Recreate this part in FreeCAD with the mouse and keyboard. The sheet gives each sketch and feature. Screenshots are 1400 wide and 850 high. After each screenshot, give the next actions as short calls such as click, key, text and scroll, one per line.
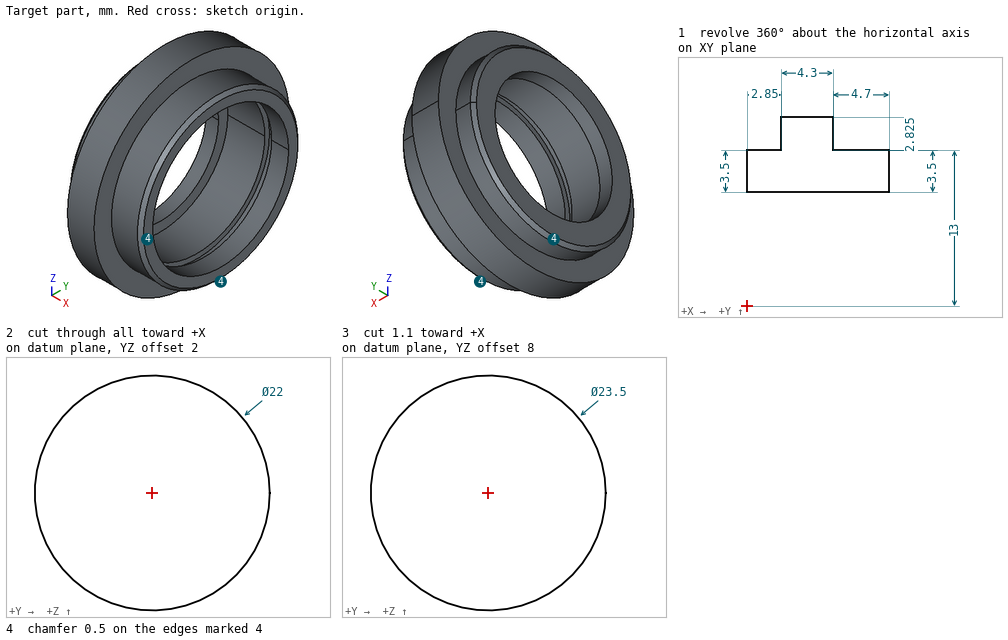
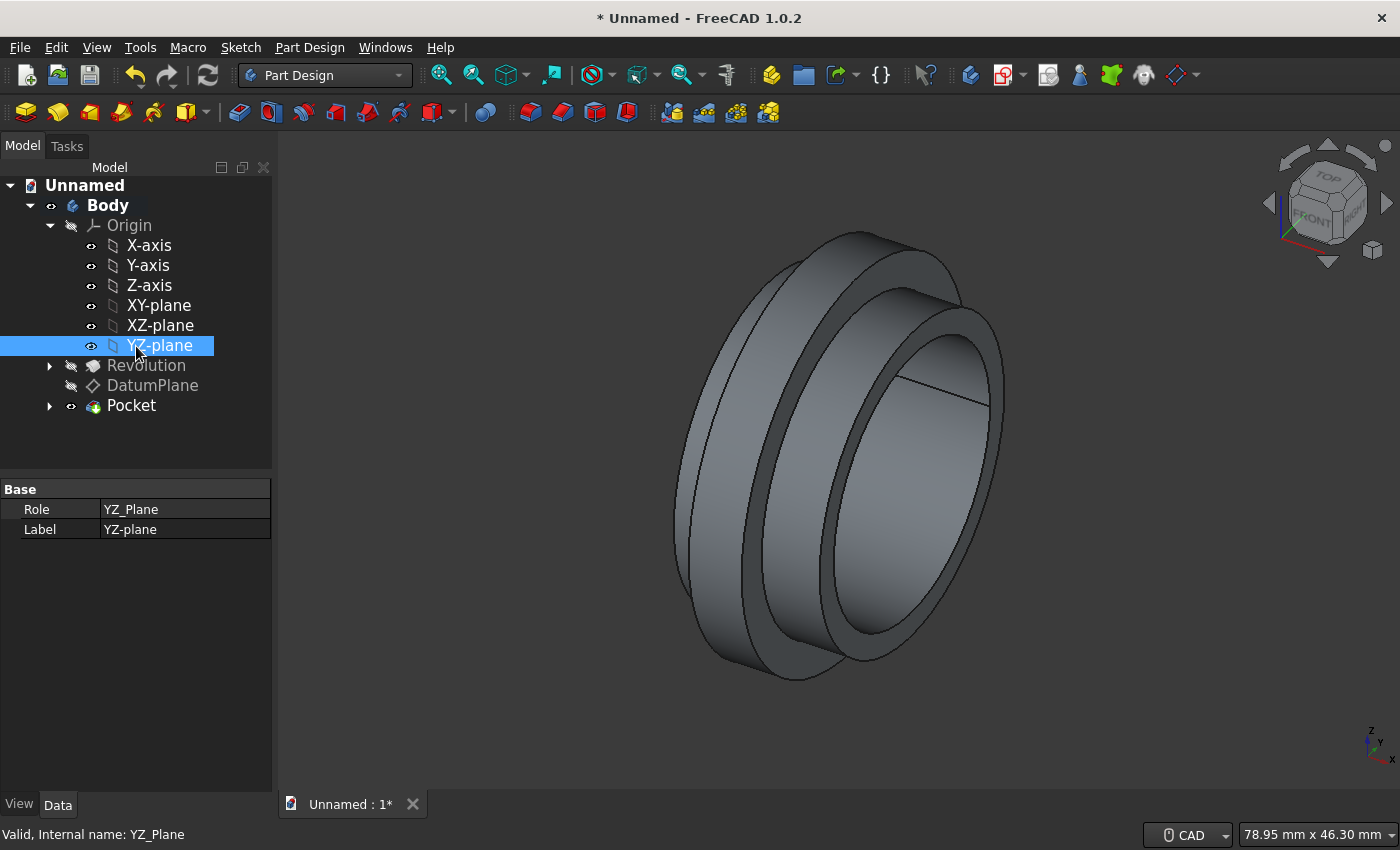
click(1176, 76)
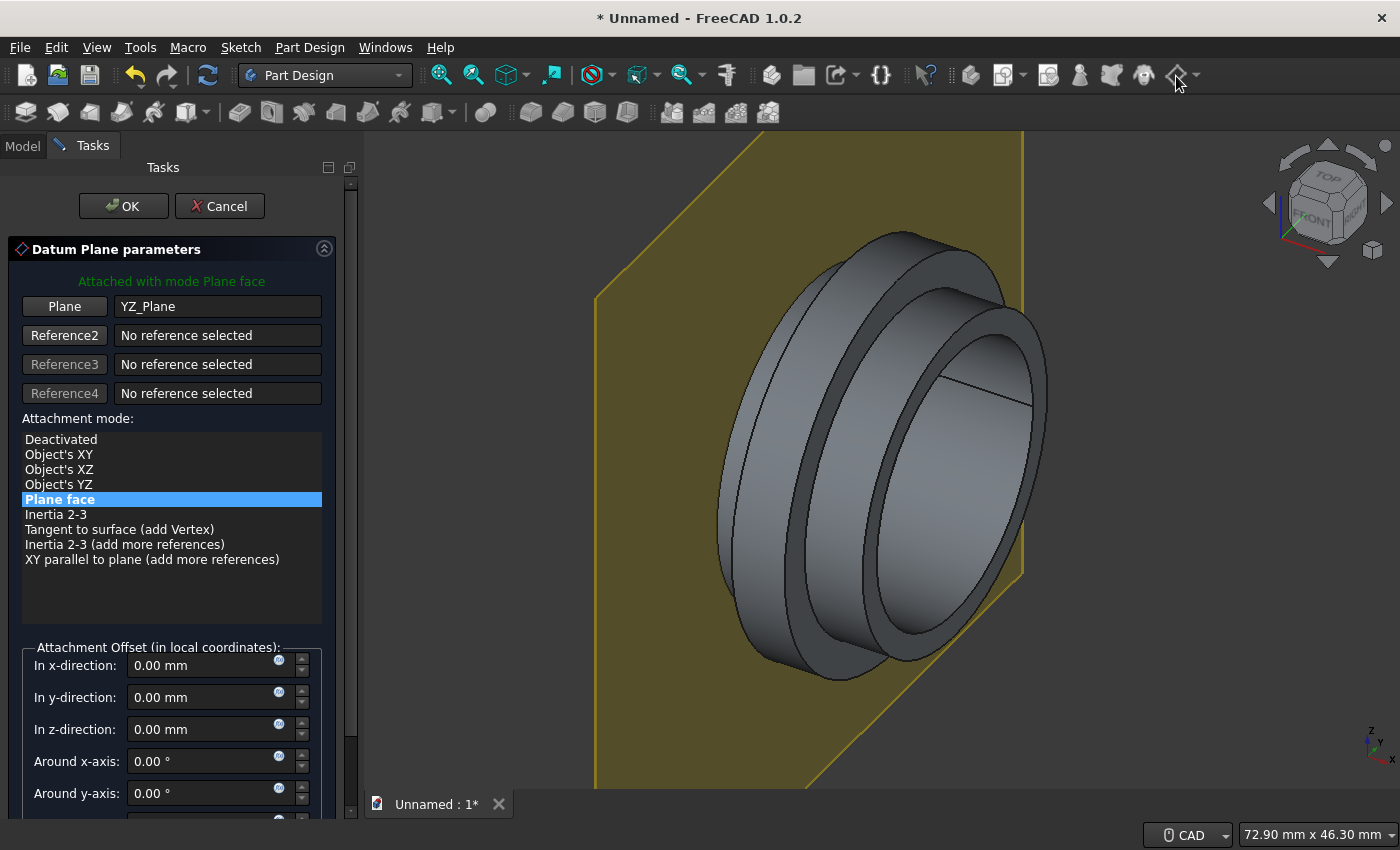
triple_click(210, 729)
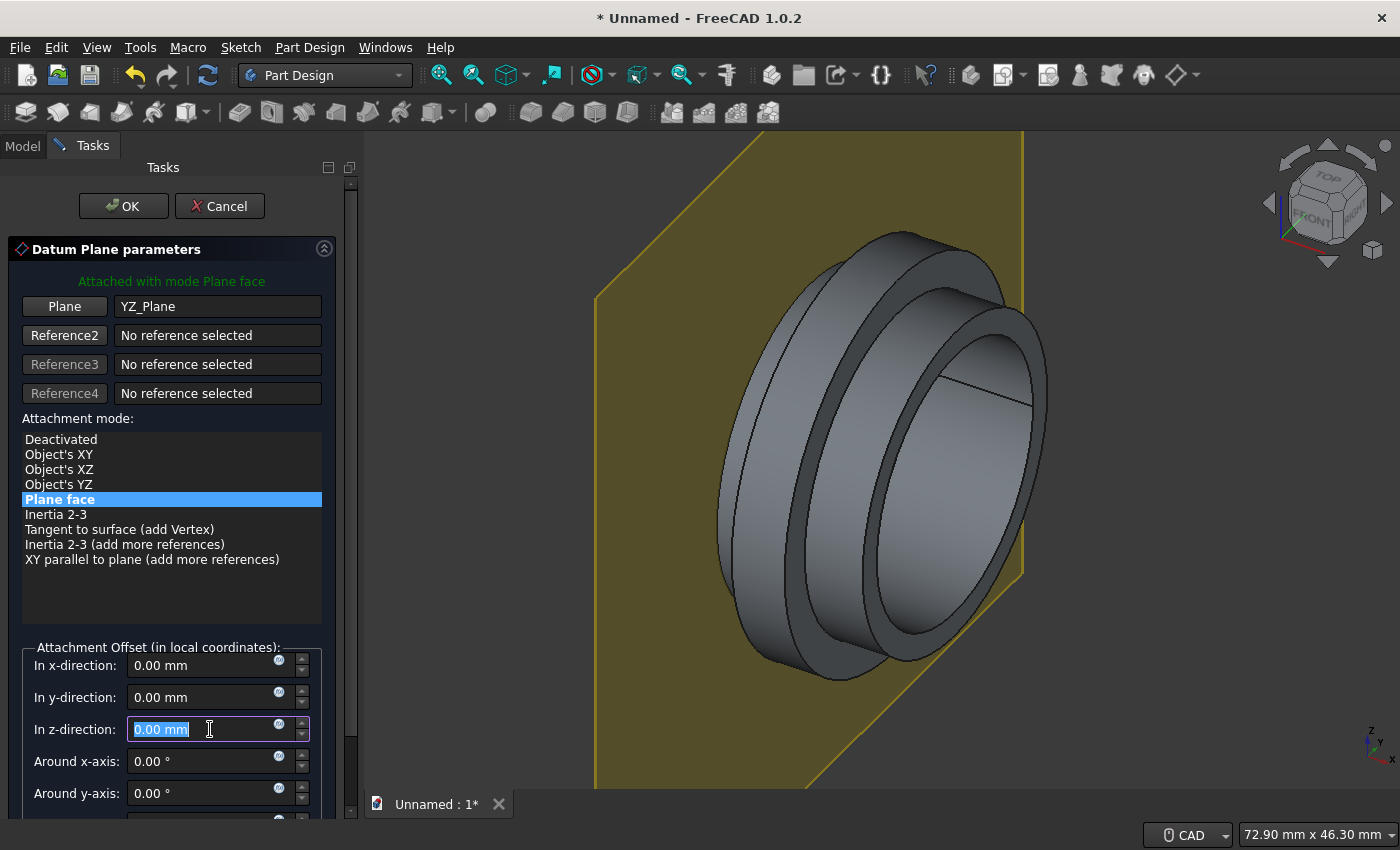
text(8)
key(Tab)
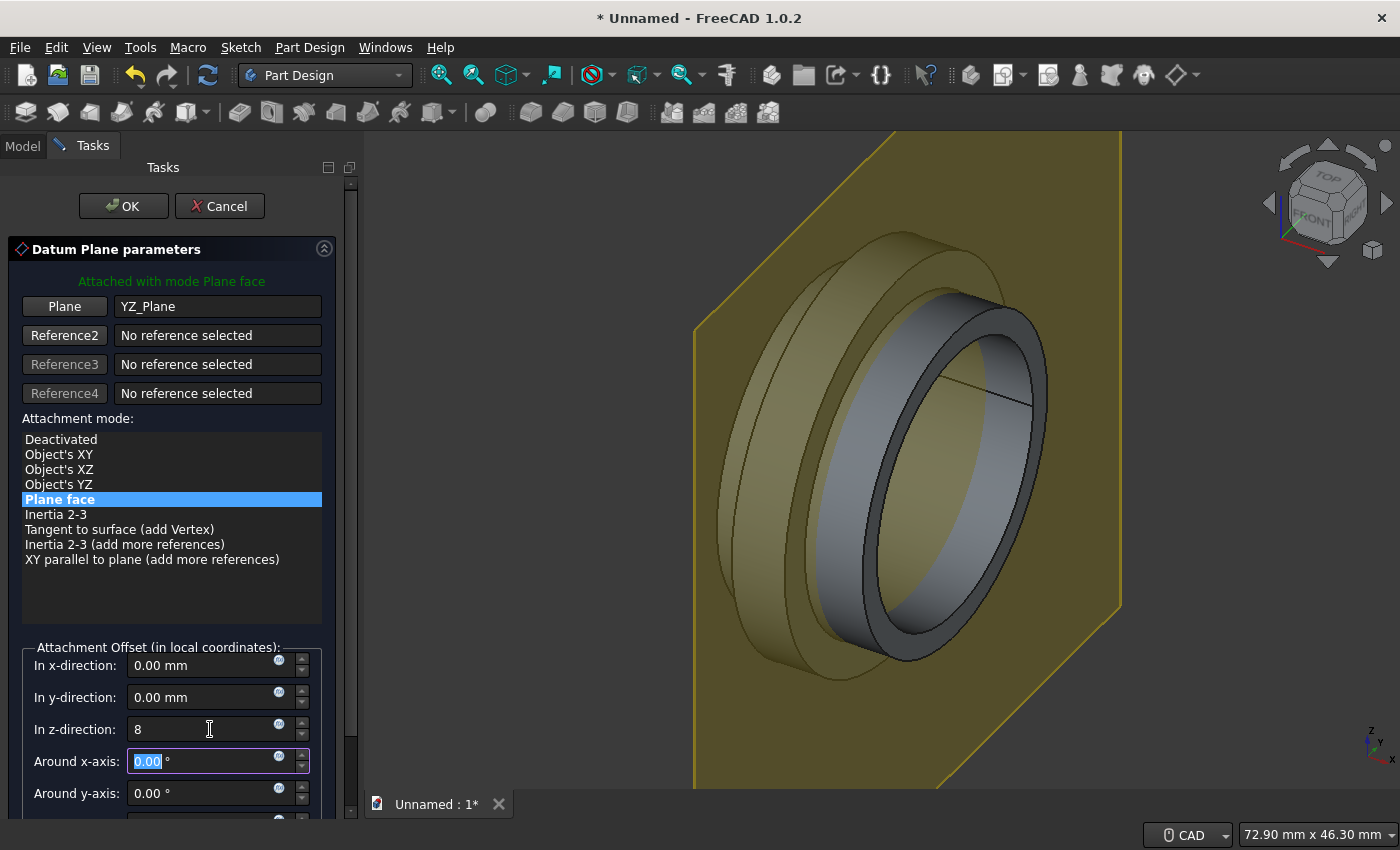
click(124, 206)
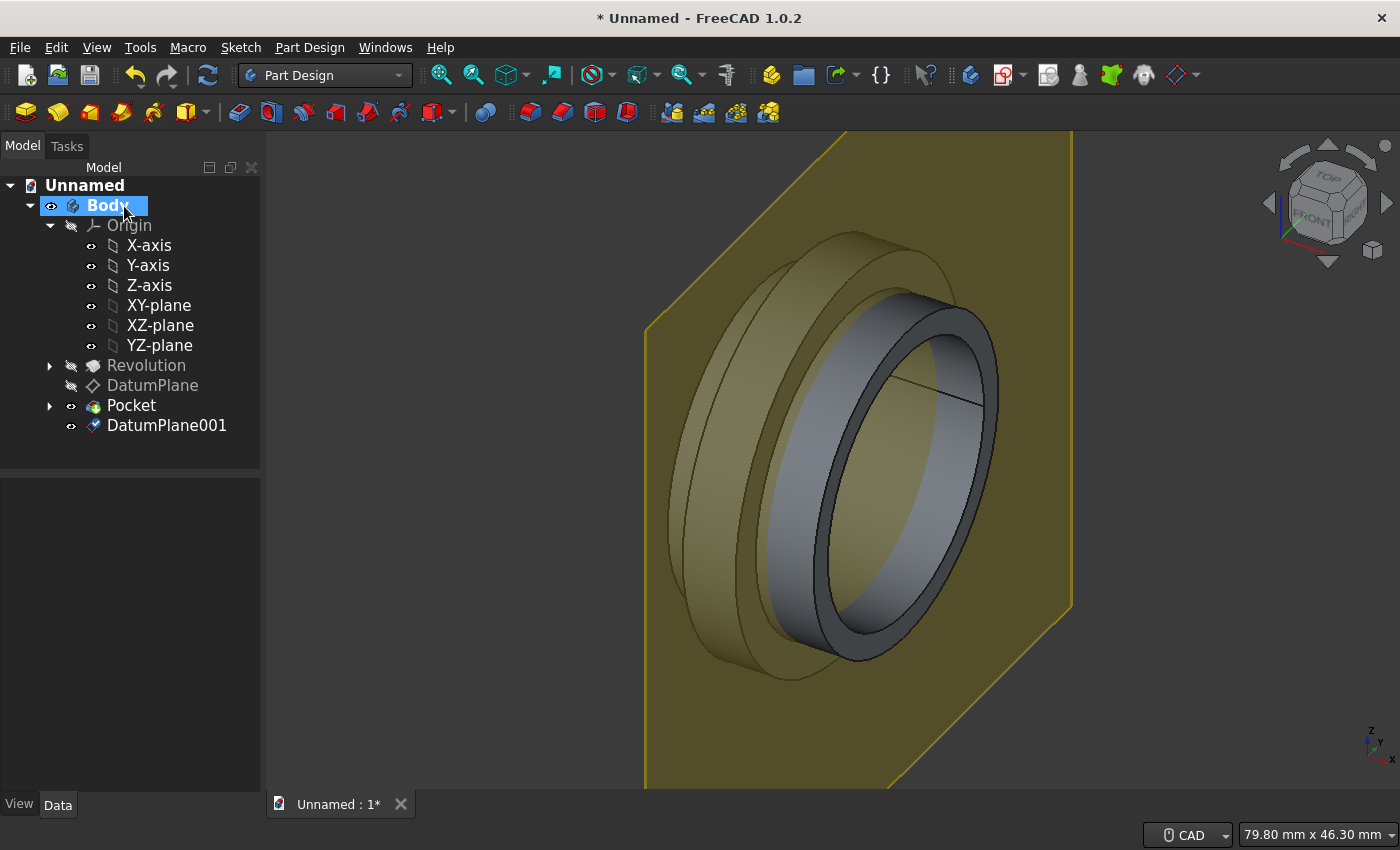
click(116, 426)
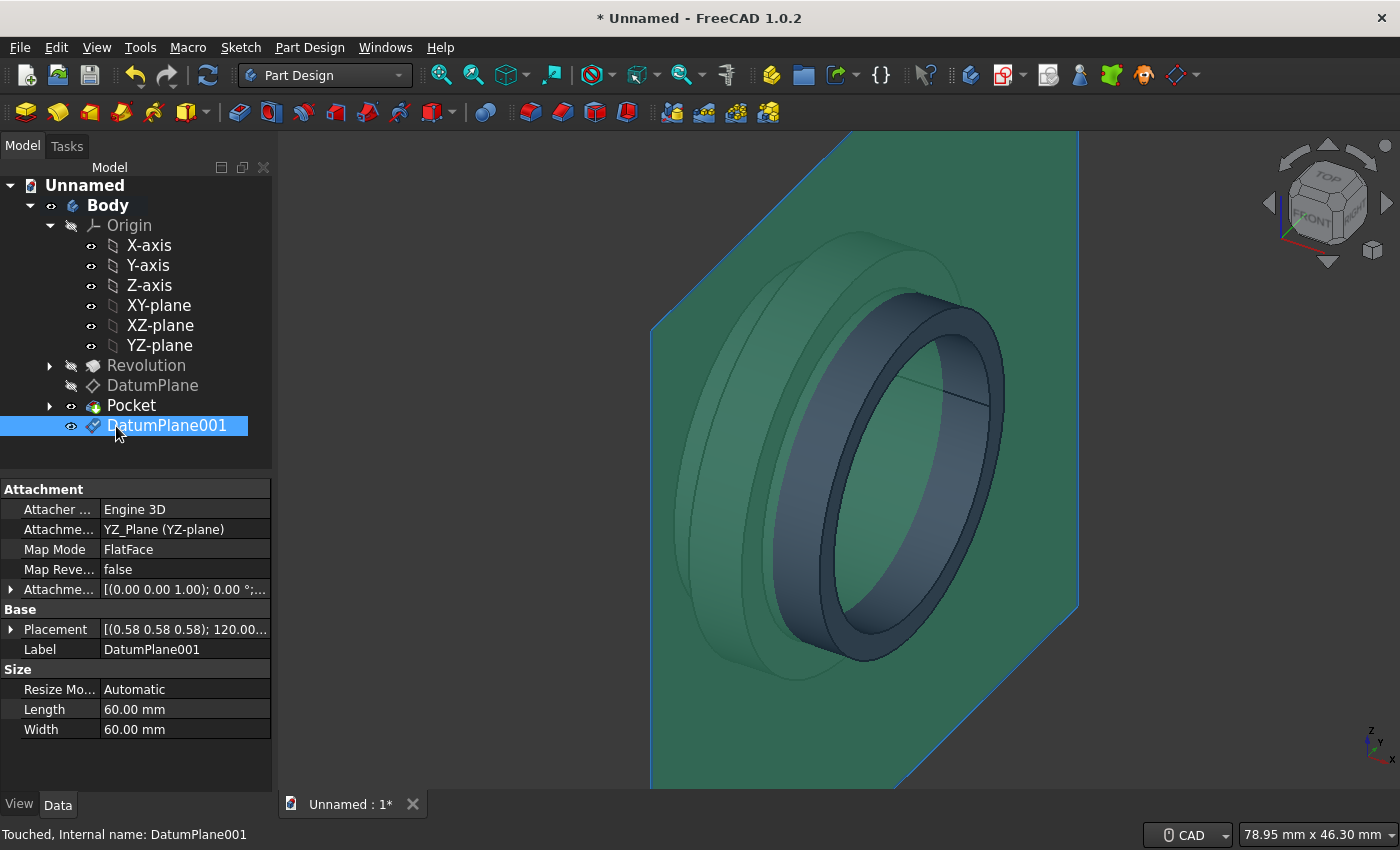
click(1004, 76)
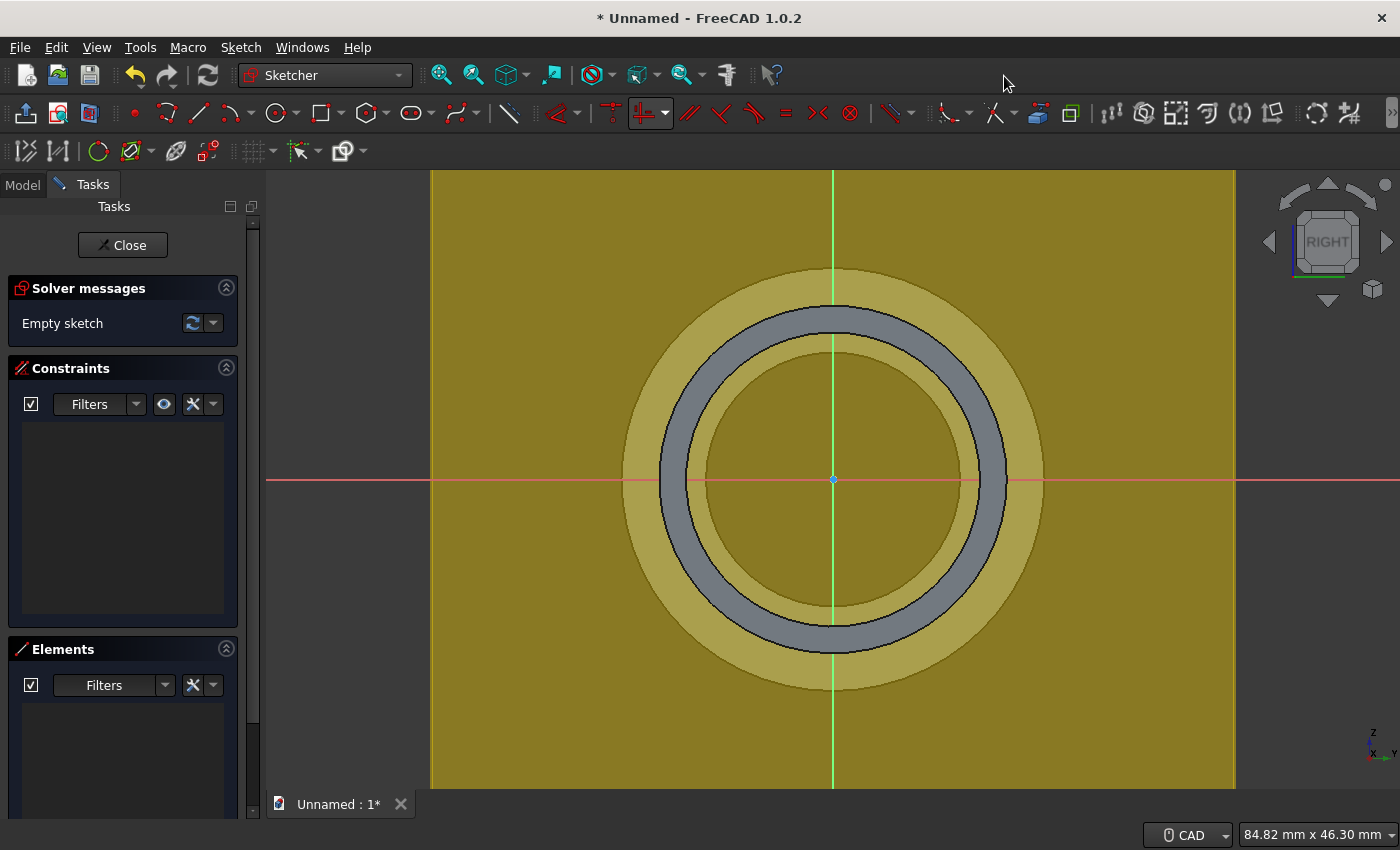
click(90, 114)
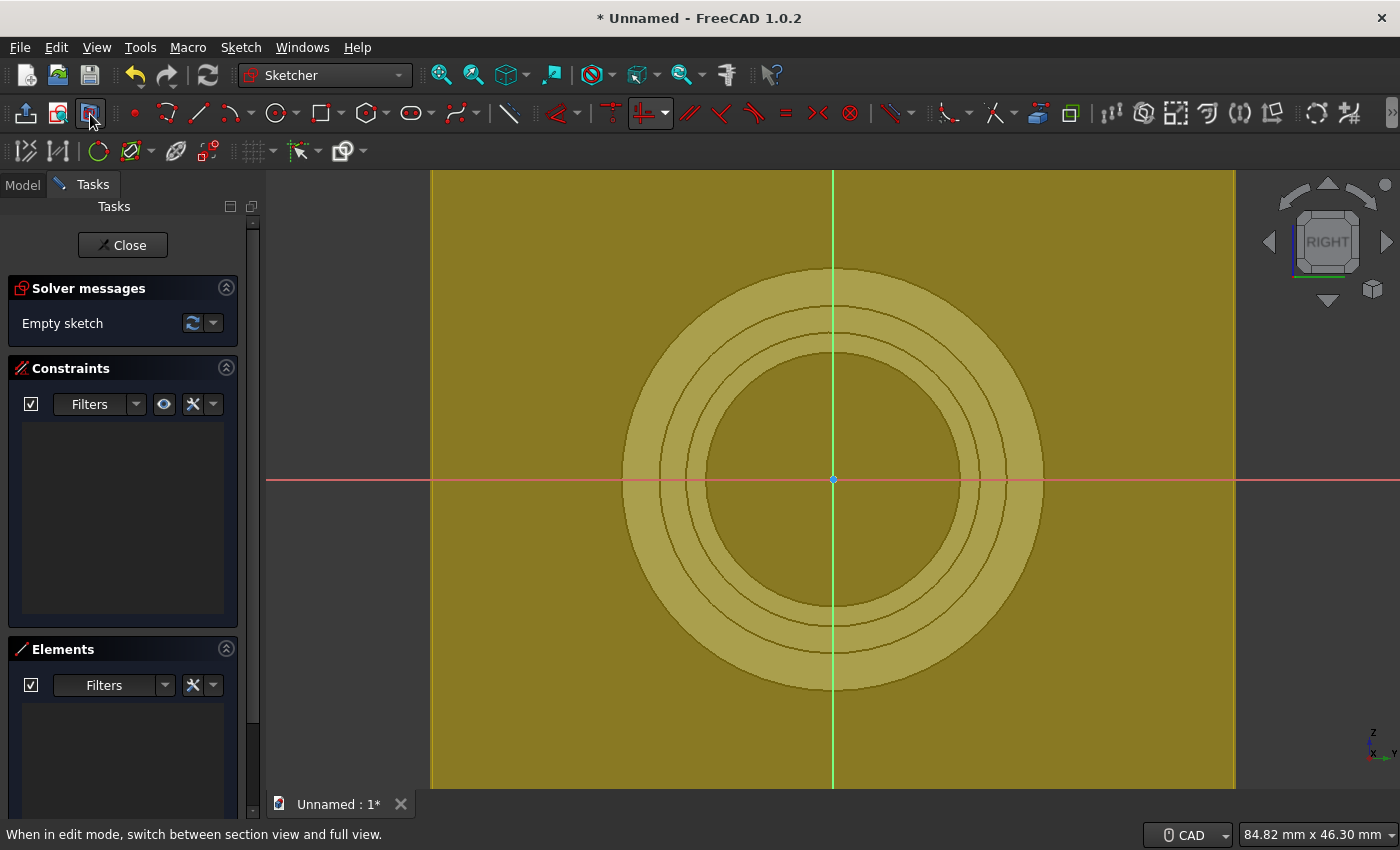
click(276, 114)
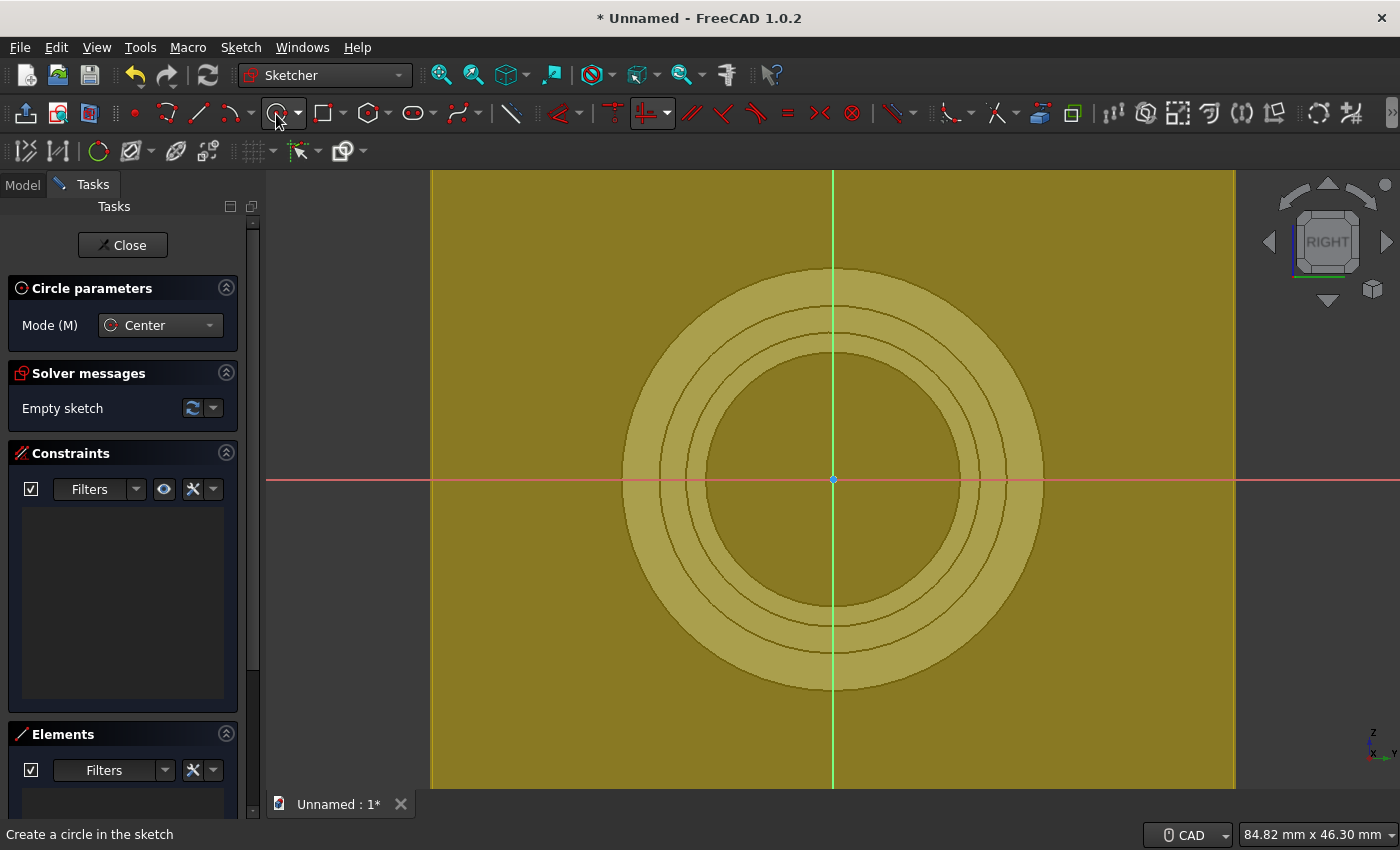
click(833, 479)
click(944, 368)
key(Escape)